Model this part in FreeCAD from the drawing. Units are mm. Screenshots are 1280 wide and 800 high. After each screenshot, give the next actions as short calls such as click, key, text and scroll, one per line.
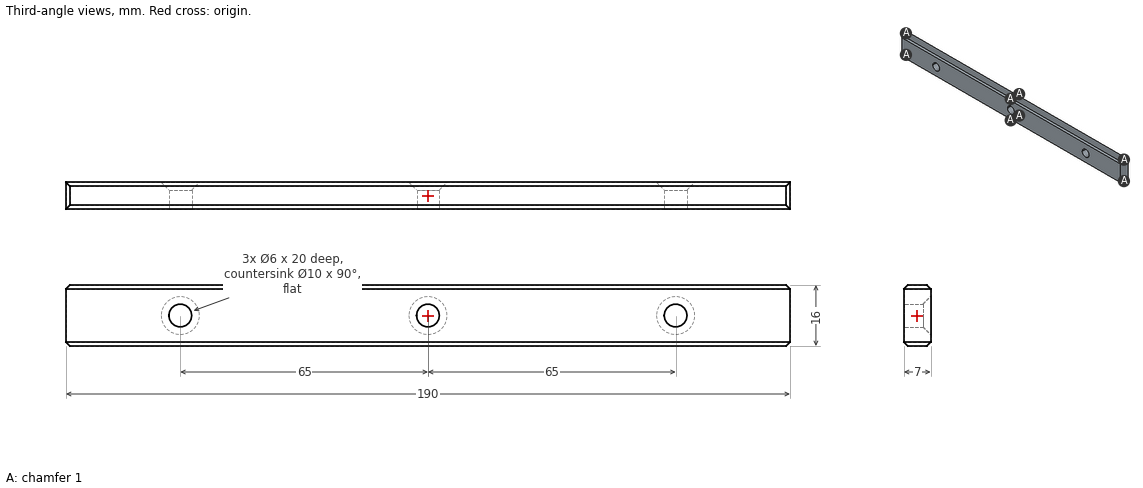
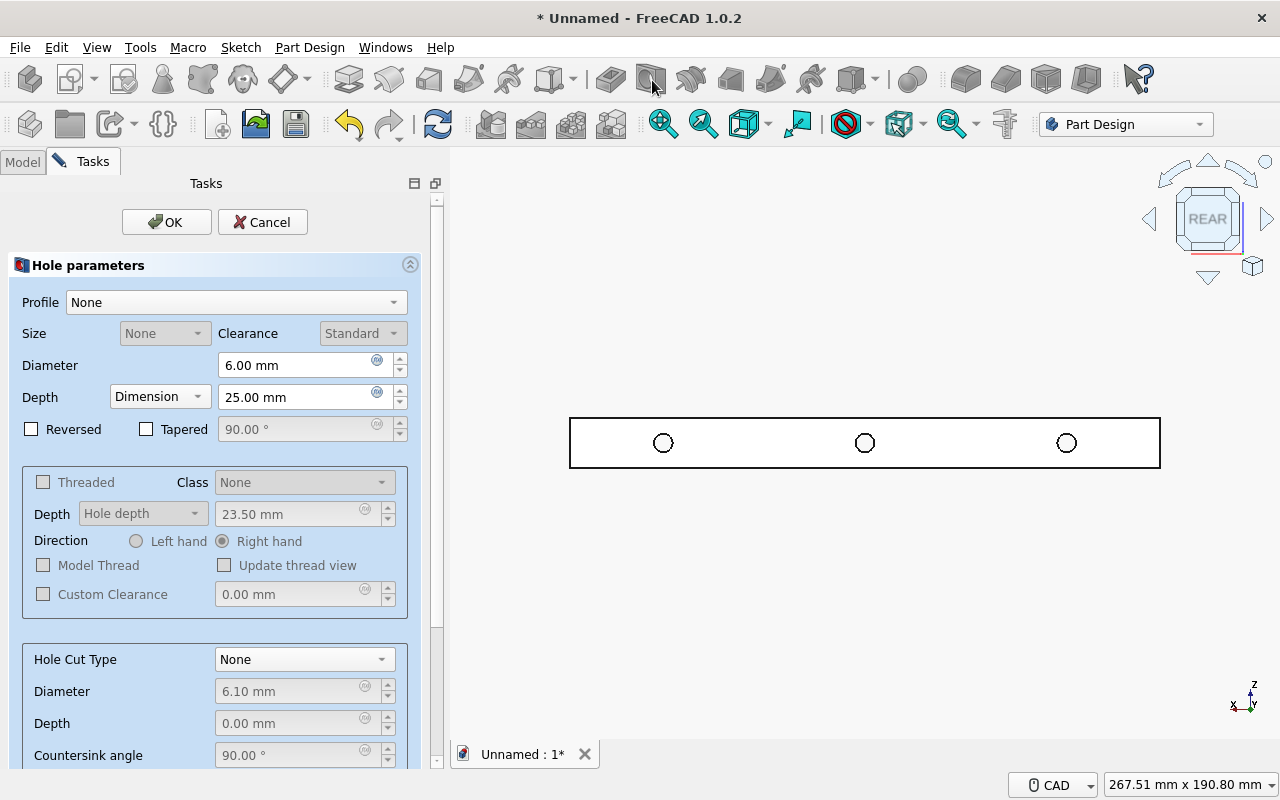
triple_click(305, 365)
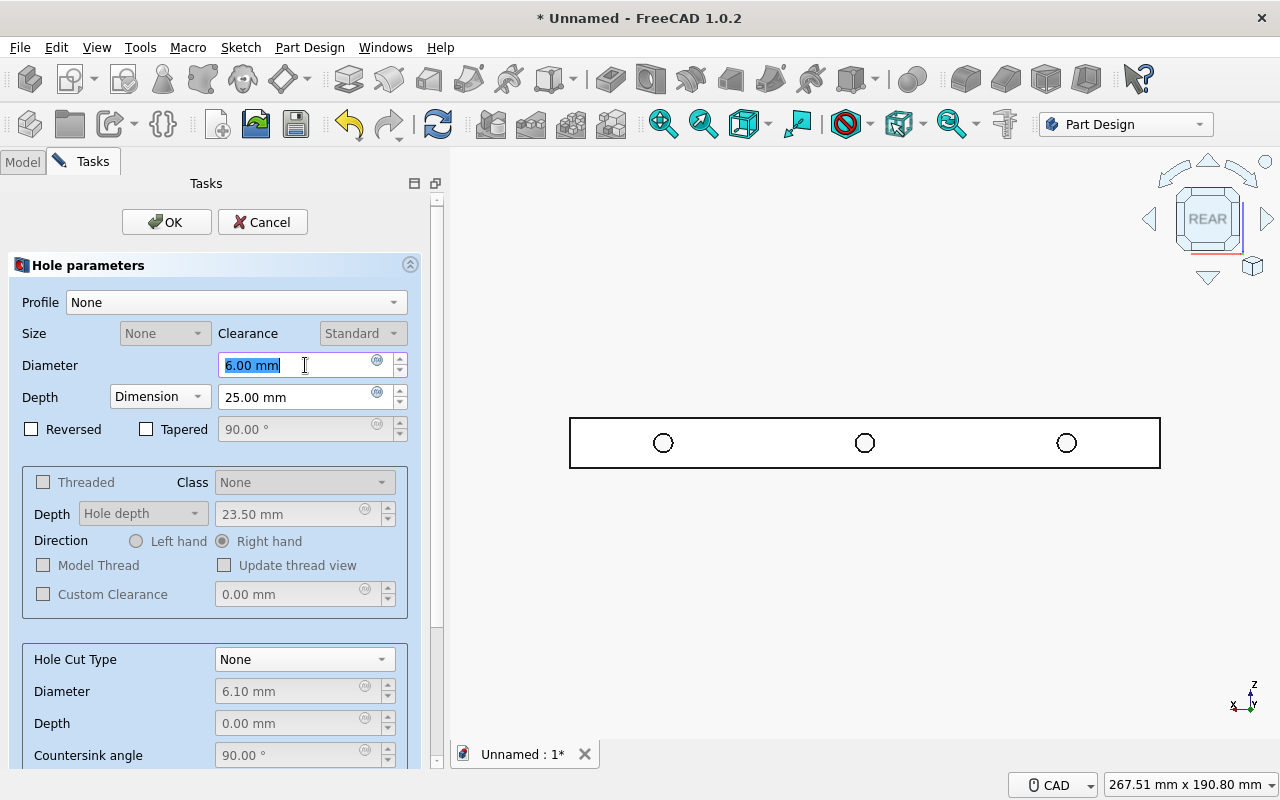
text(6)
key(Tab)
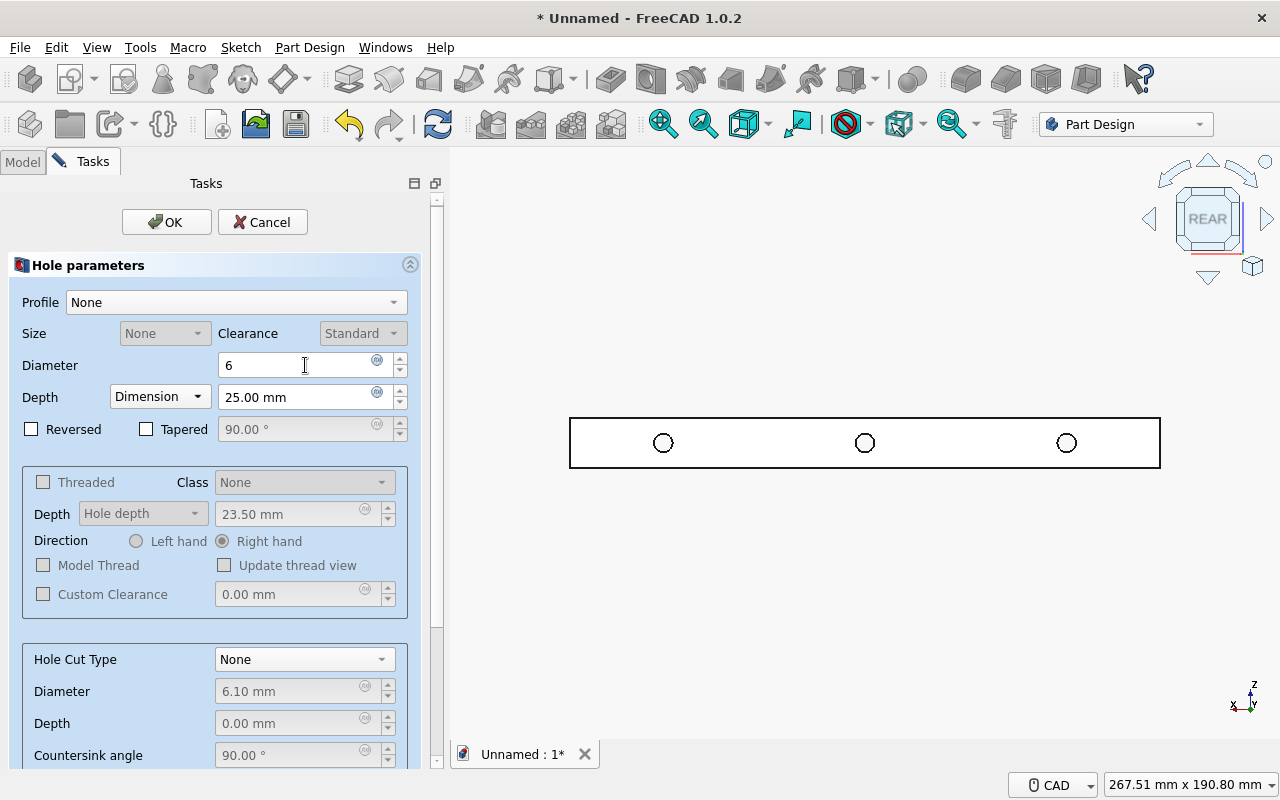
triple_click(305, 397)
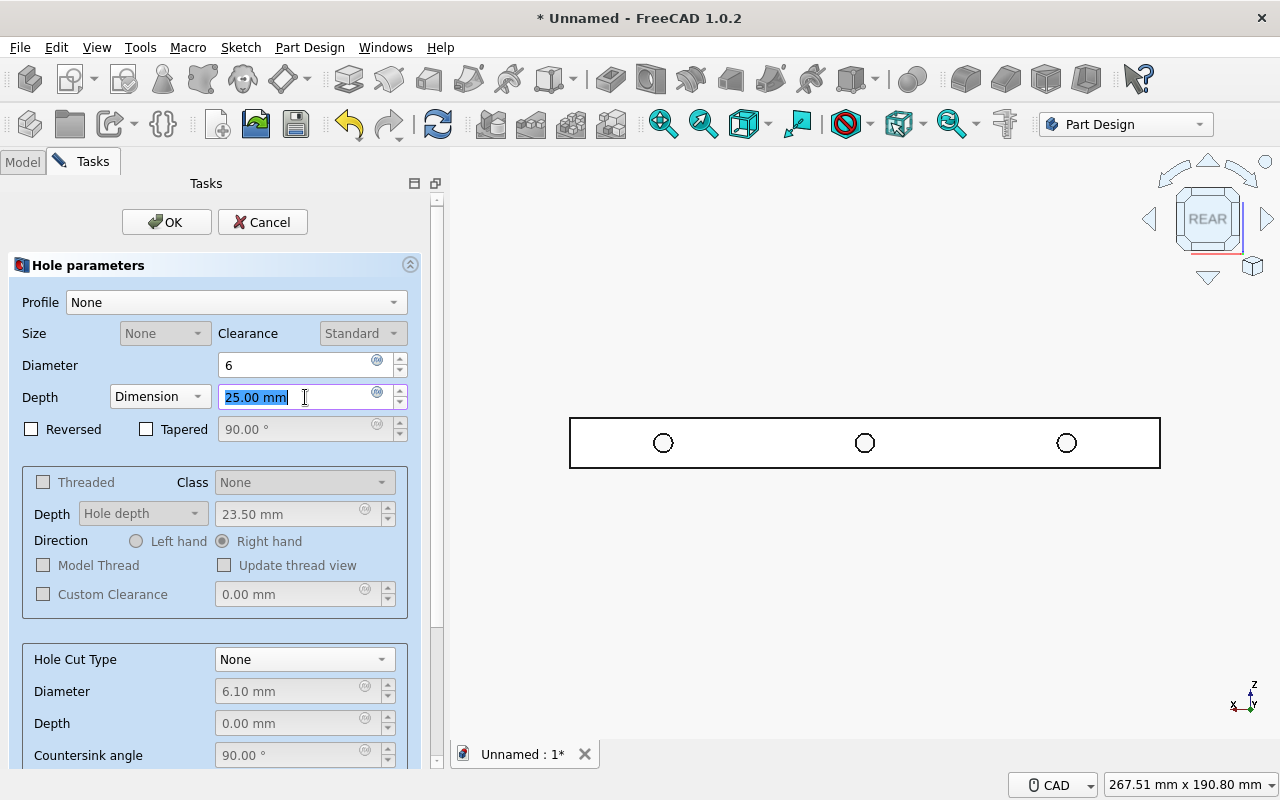
text(20)
key(Tab)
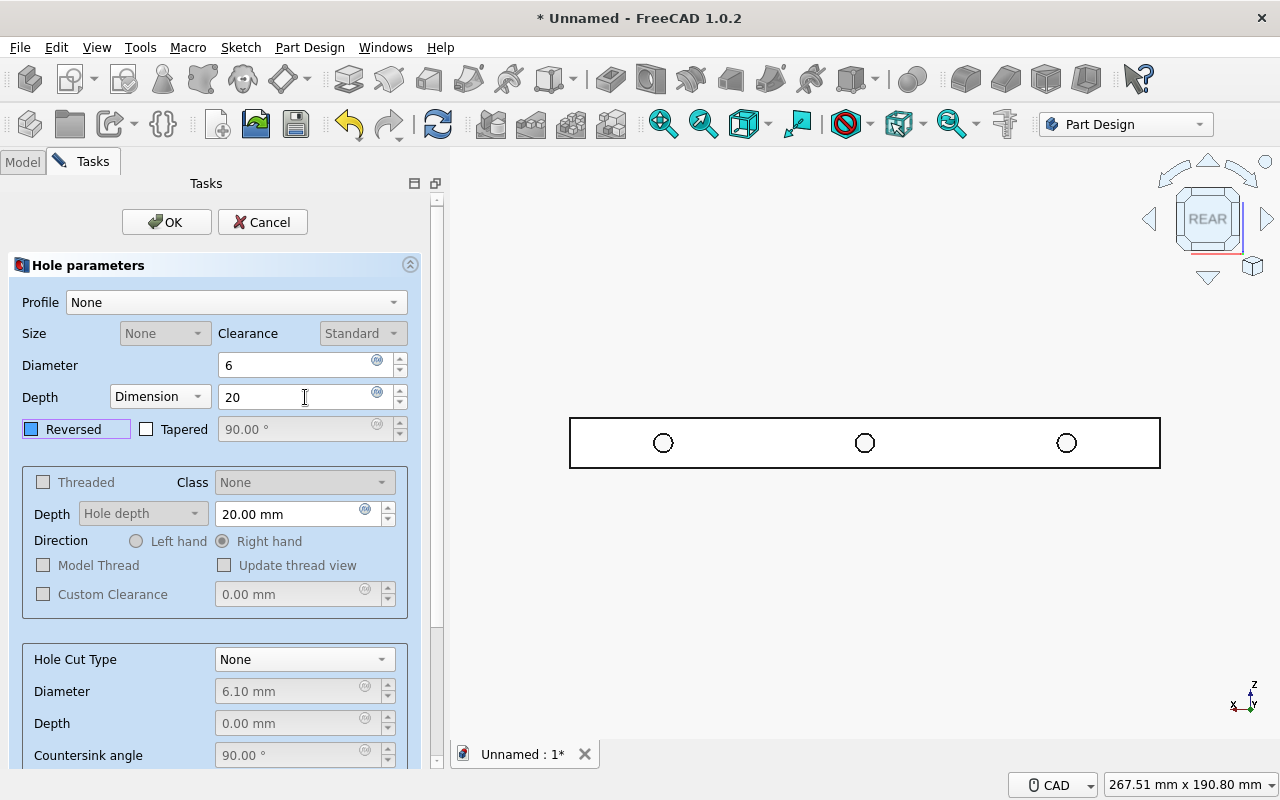
click(306, 660)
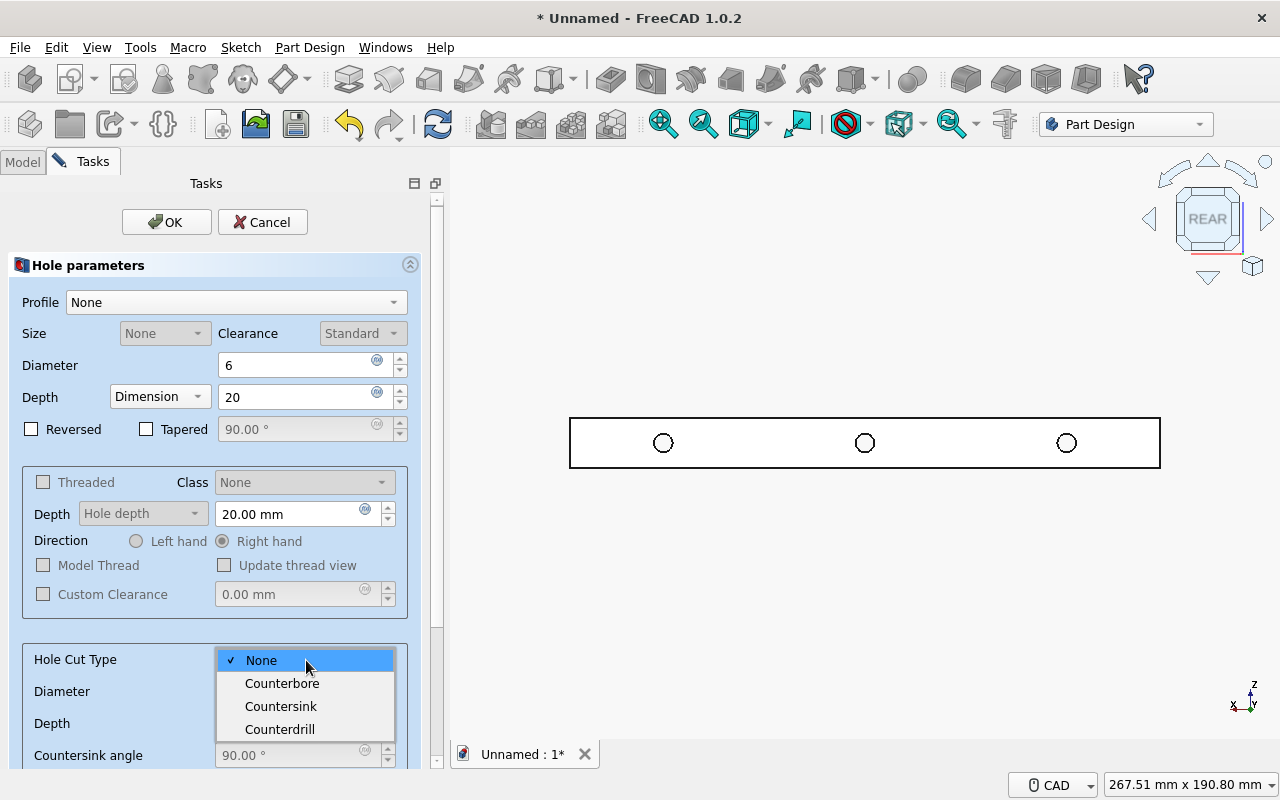
click(304, 706)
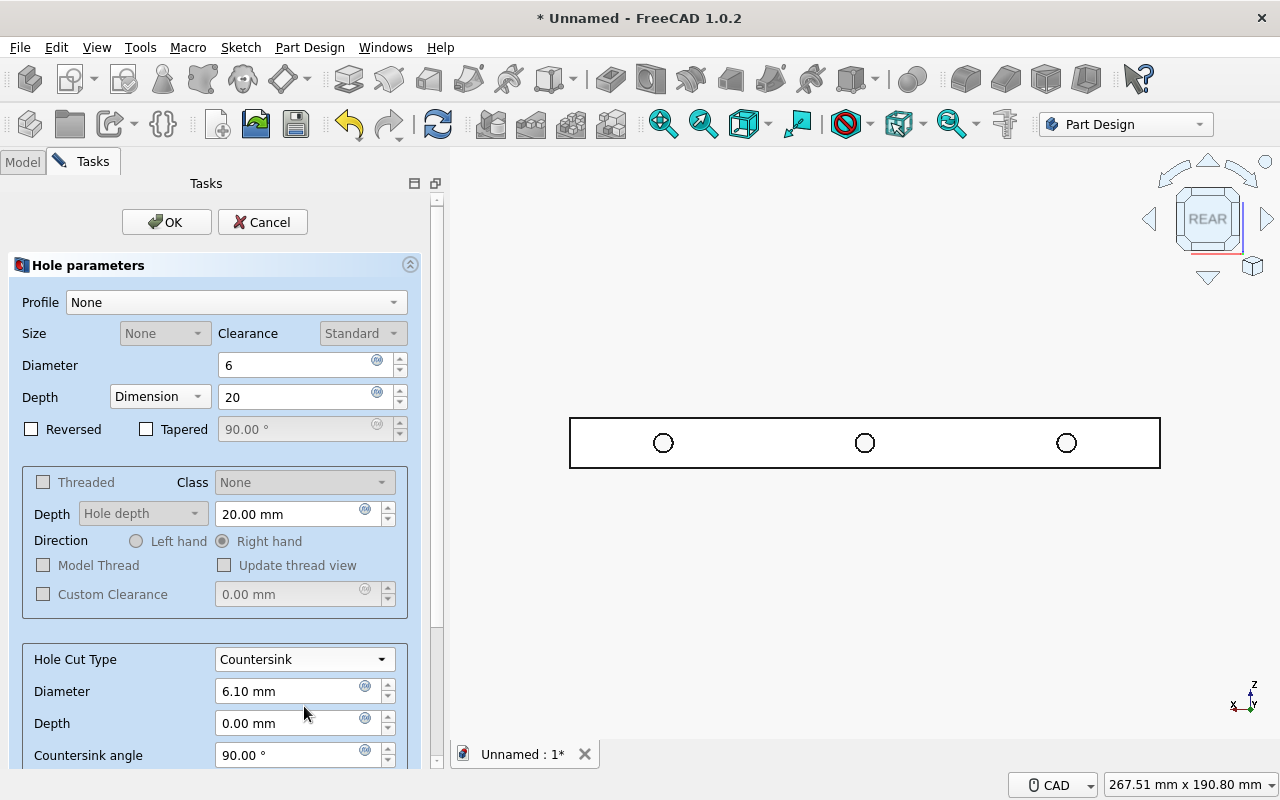
triple_click(298, 691)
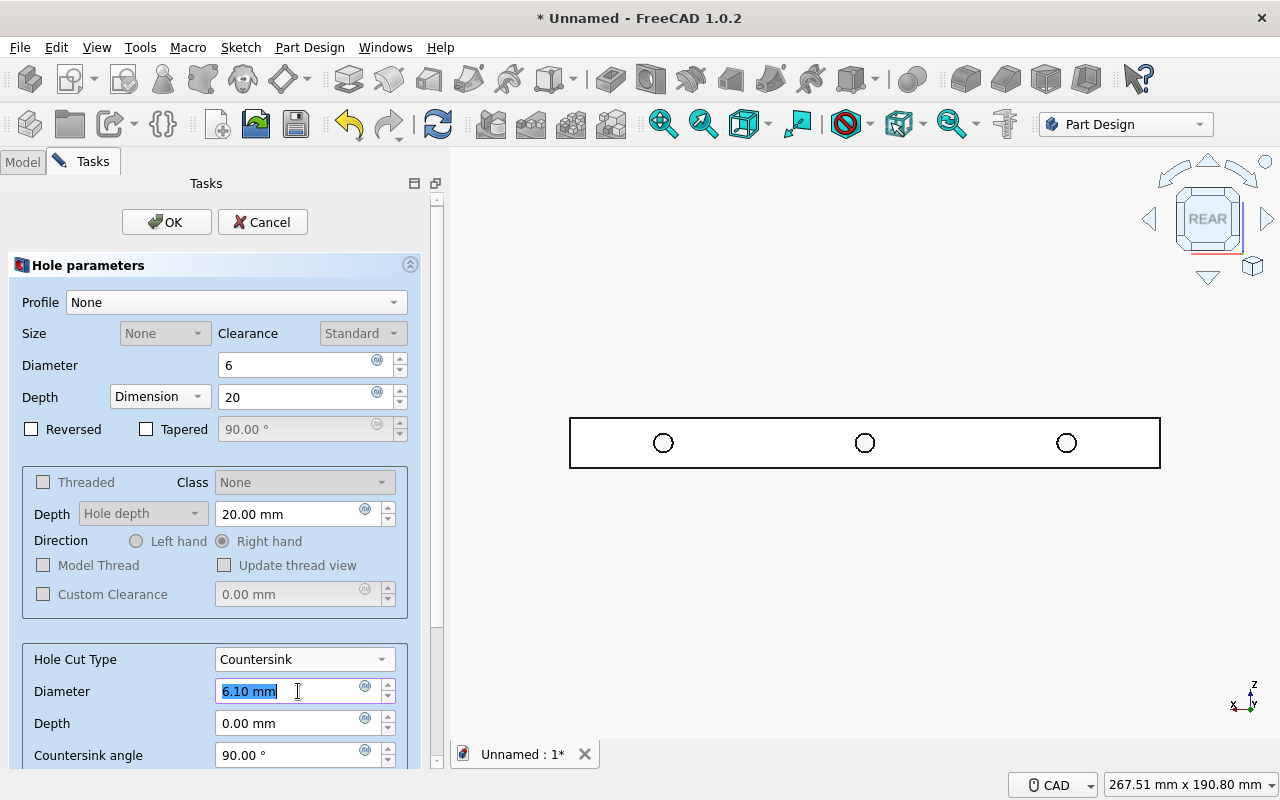
text(10)
key(Tab)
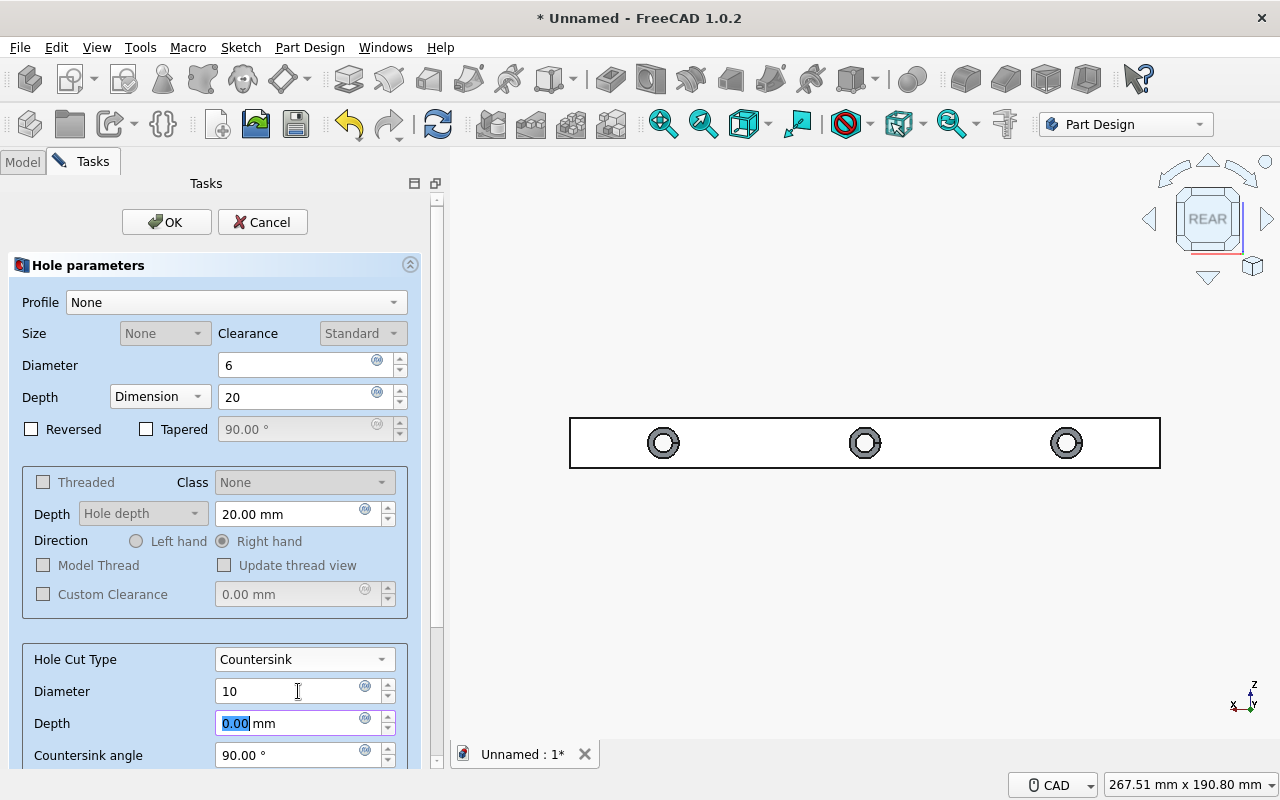
scroll(437, 480, down, 3)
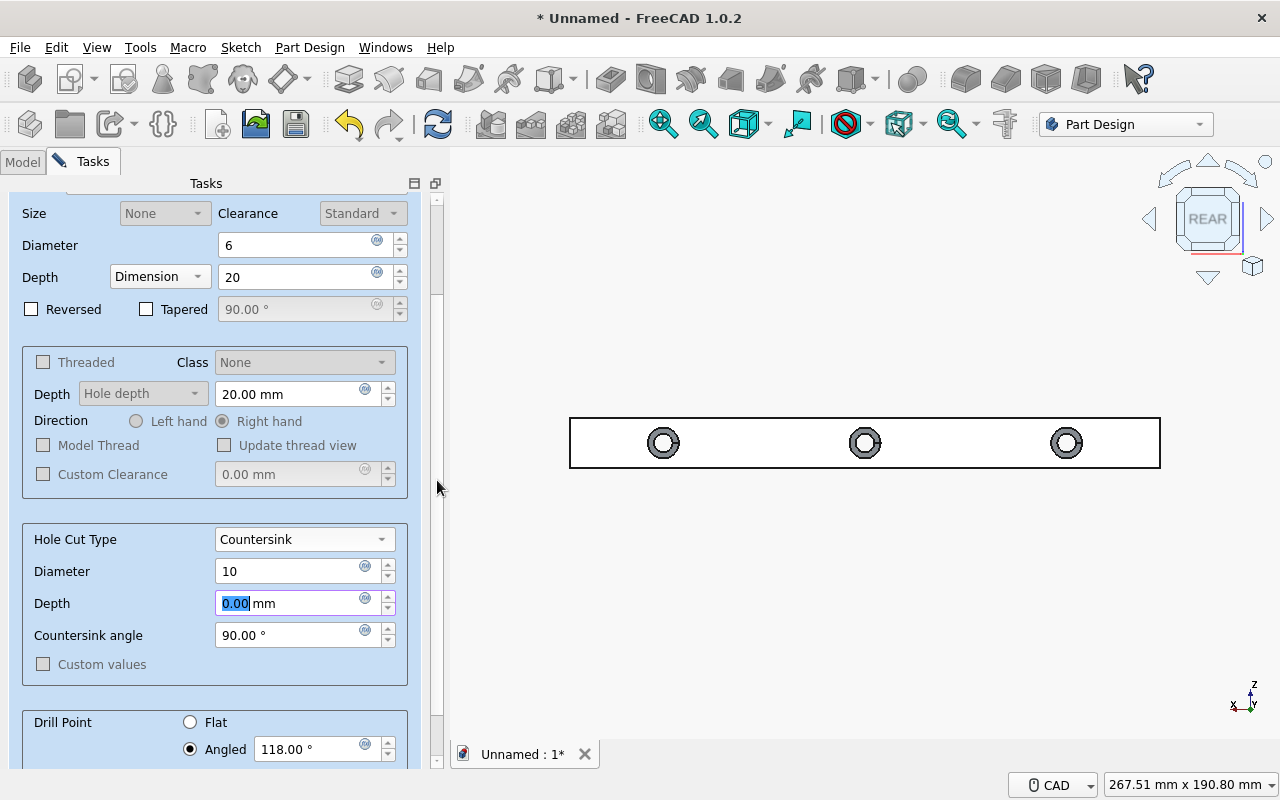
click(191, 669)